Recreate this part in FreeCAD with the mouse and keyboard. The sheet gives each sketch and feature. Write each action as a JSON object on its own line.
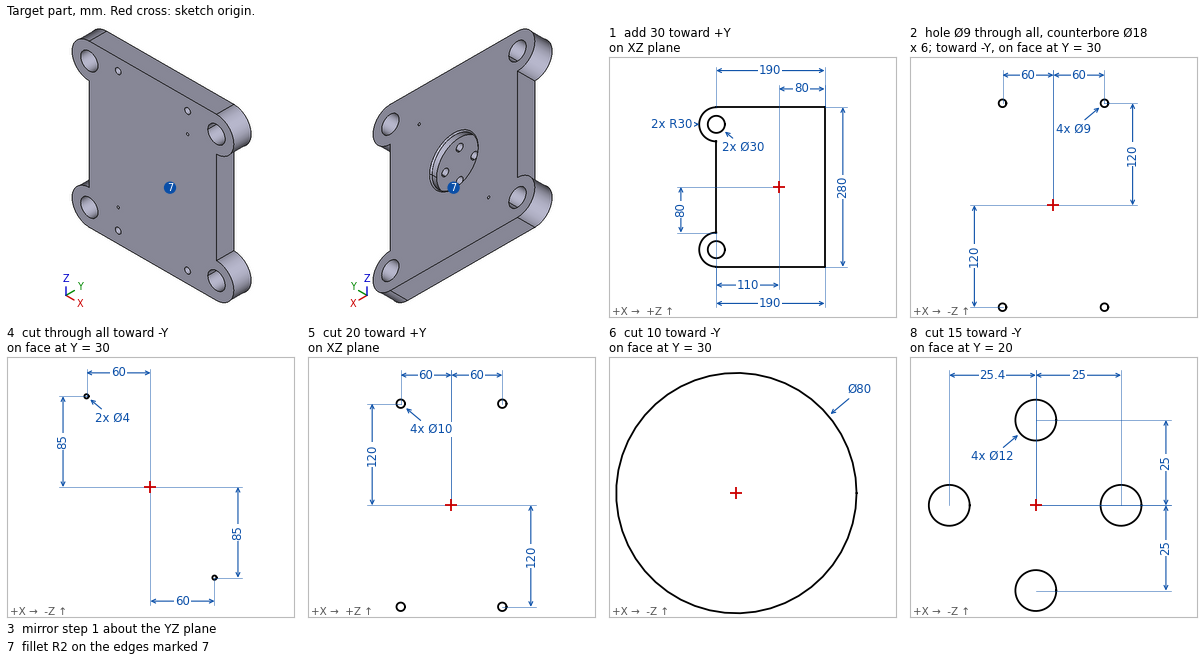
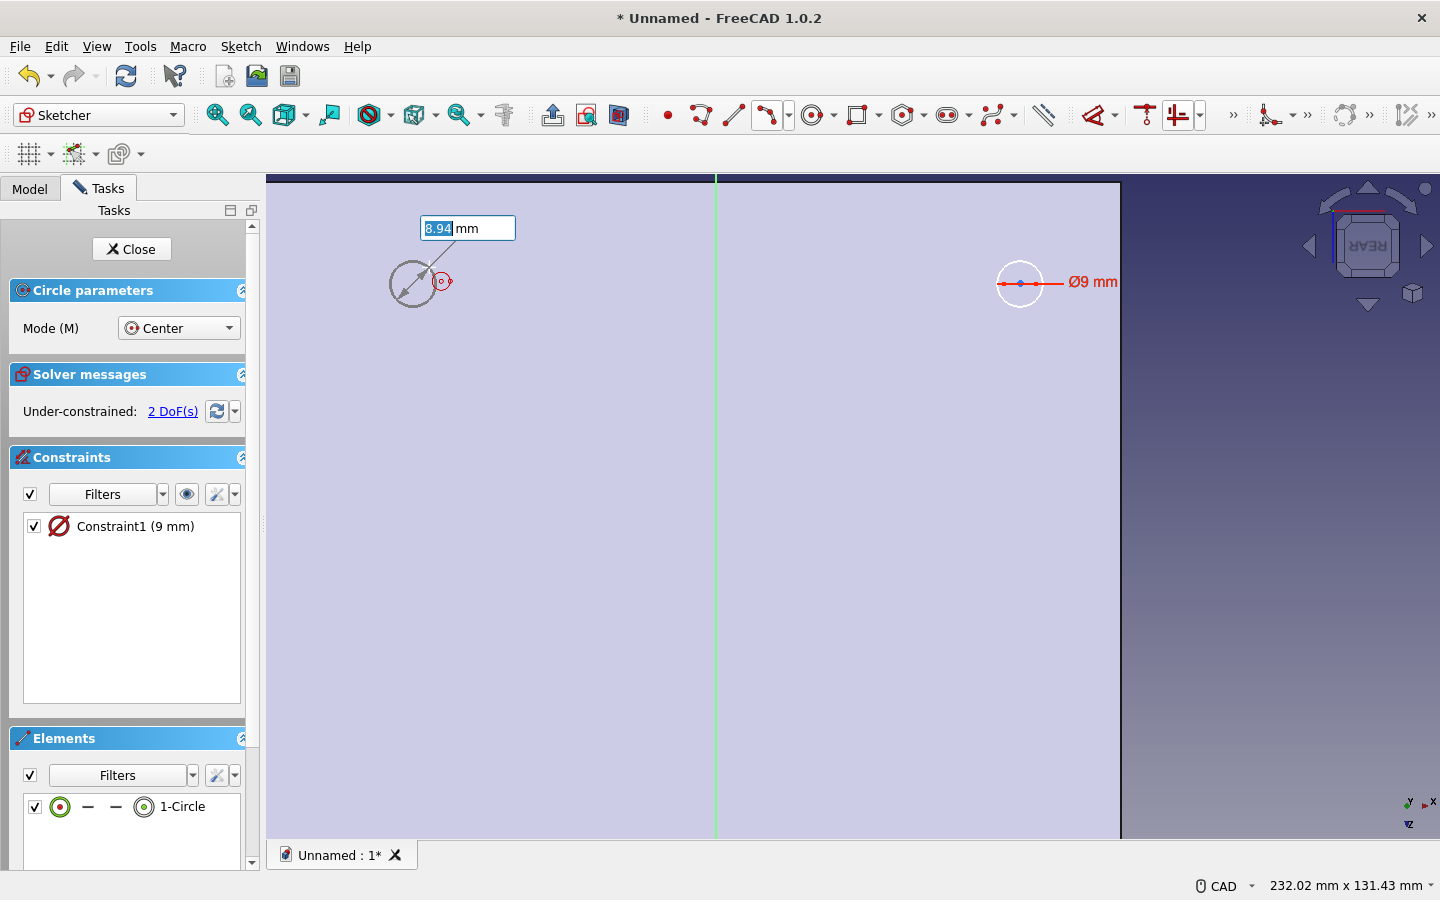
{"action": "type", "text": "9"}
{"action": "key", "text": "Return"}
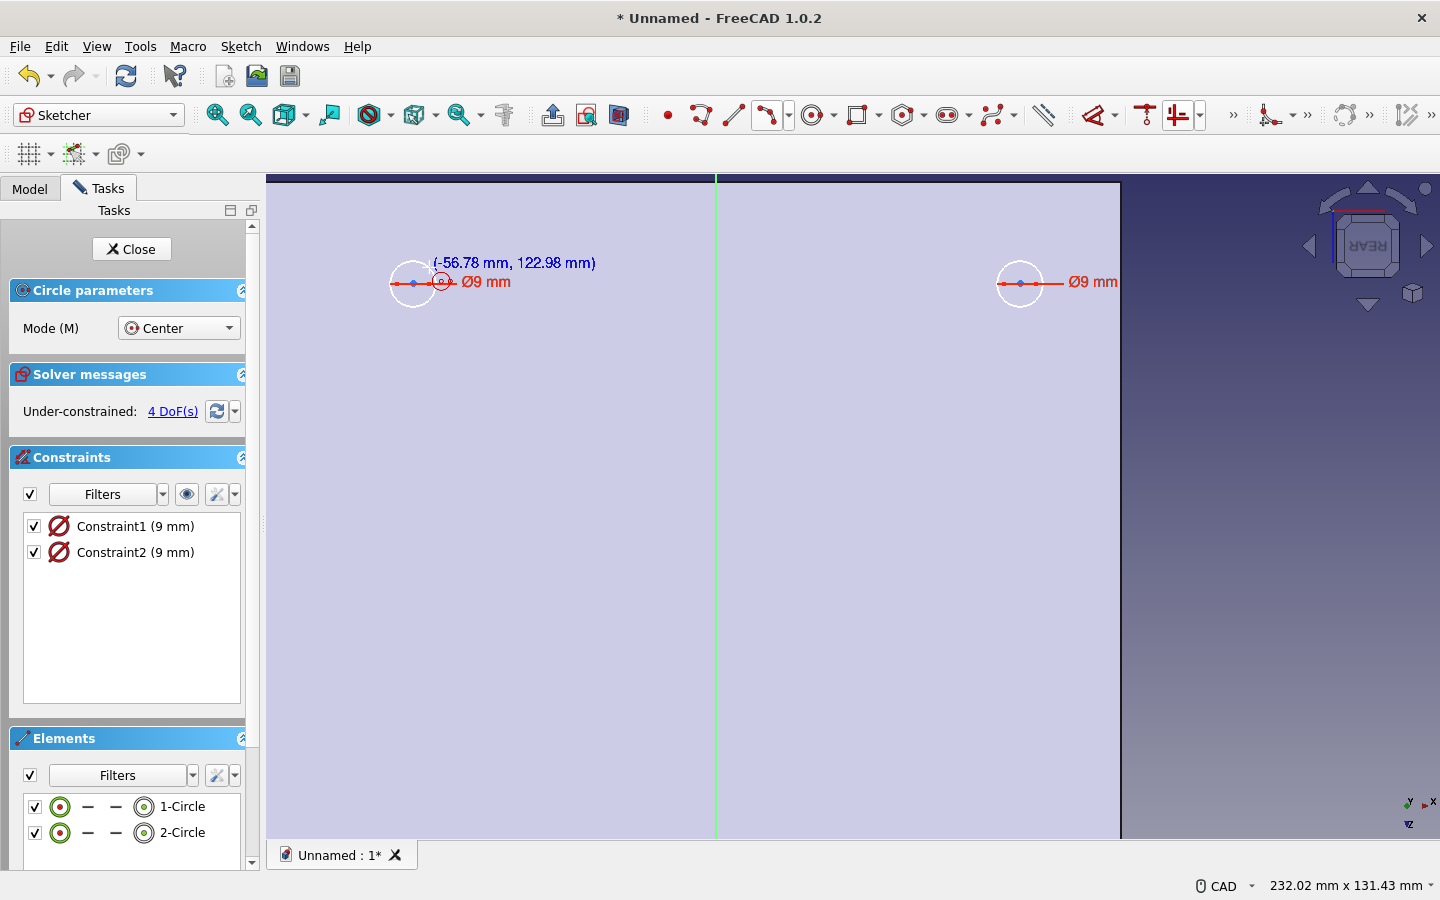
{"action": "scroll", "coordinate": [824, 283], "scroll_direction": "down", "scroll_amount": 5}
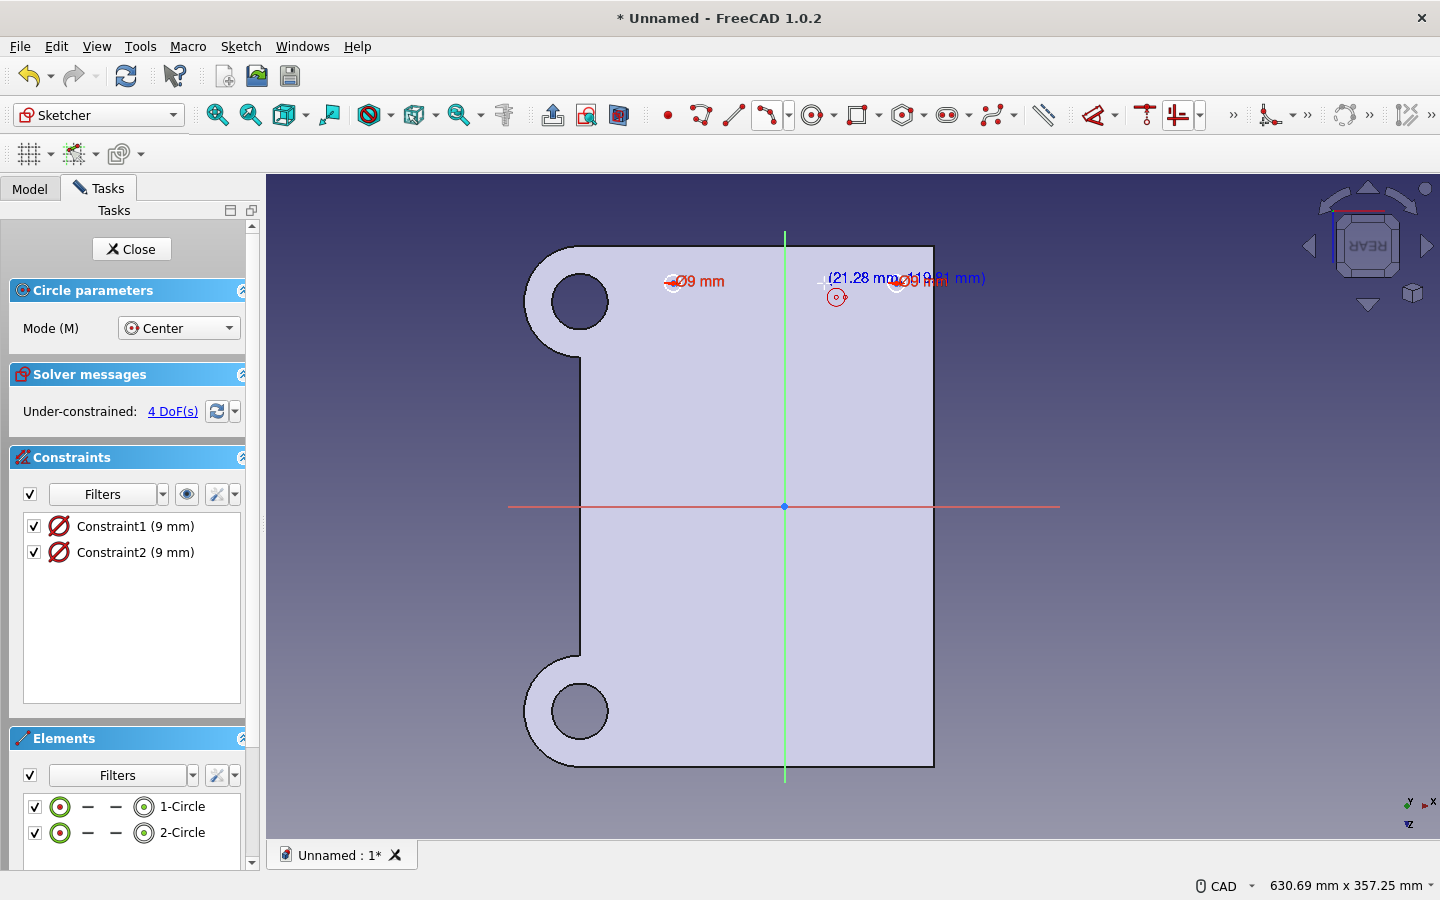
{"action": "scroll", "coordinate": [673, 730], "scroll_direction": "up", "scroll_amount": 5}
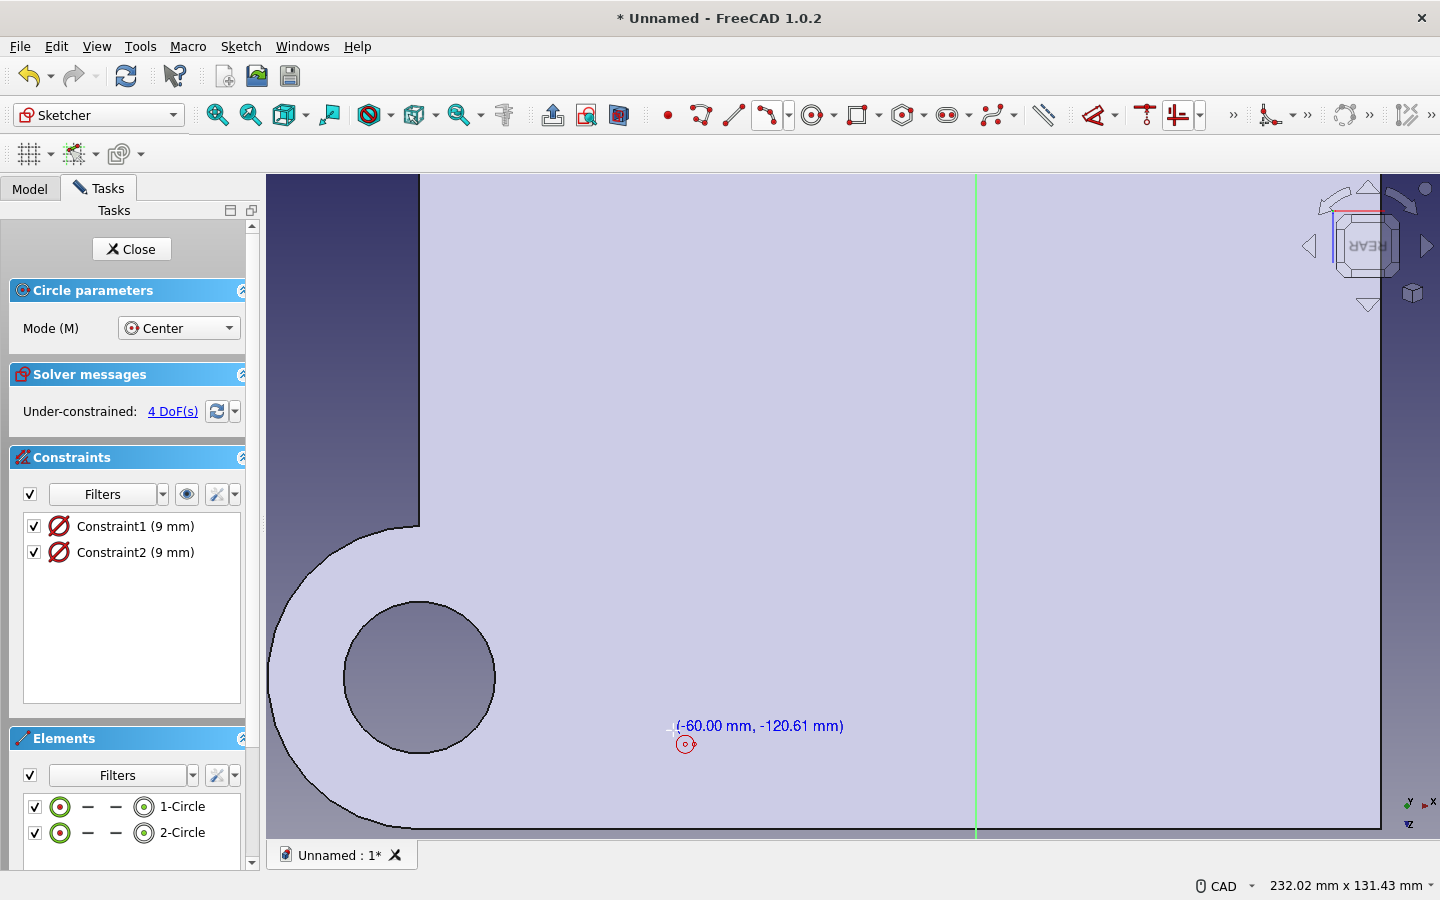
{"action": "left_click", "coordinate": [672, 728]}
{"action": "mouse_move", "coordinate": [689, 712]}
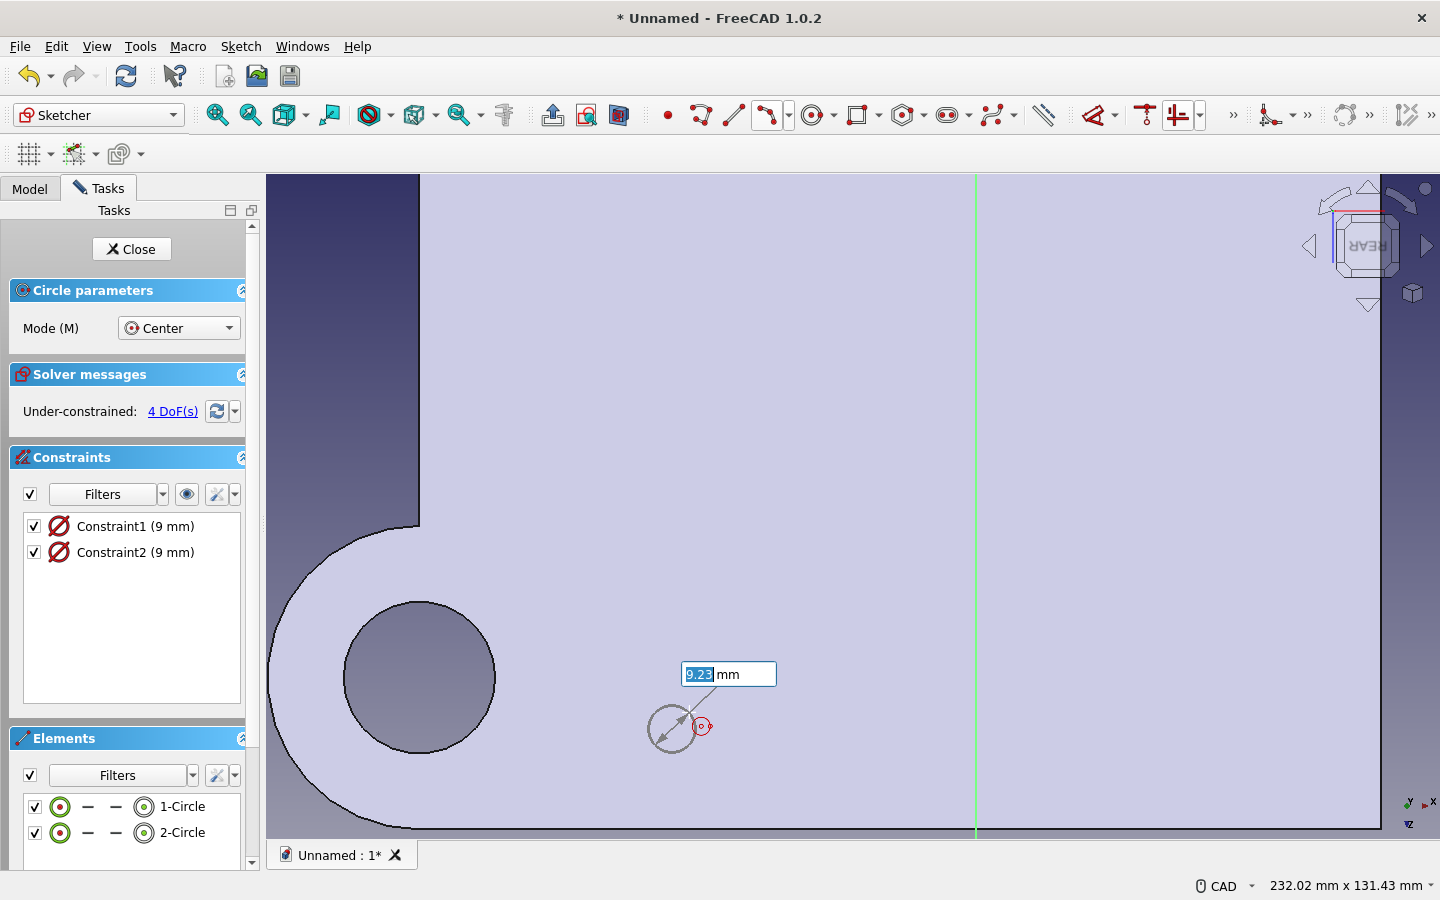
{"action": "type", "text": "9"}
{"action": "key", "text": "Return"}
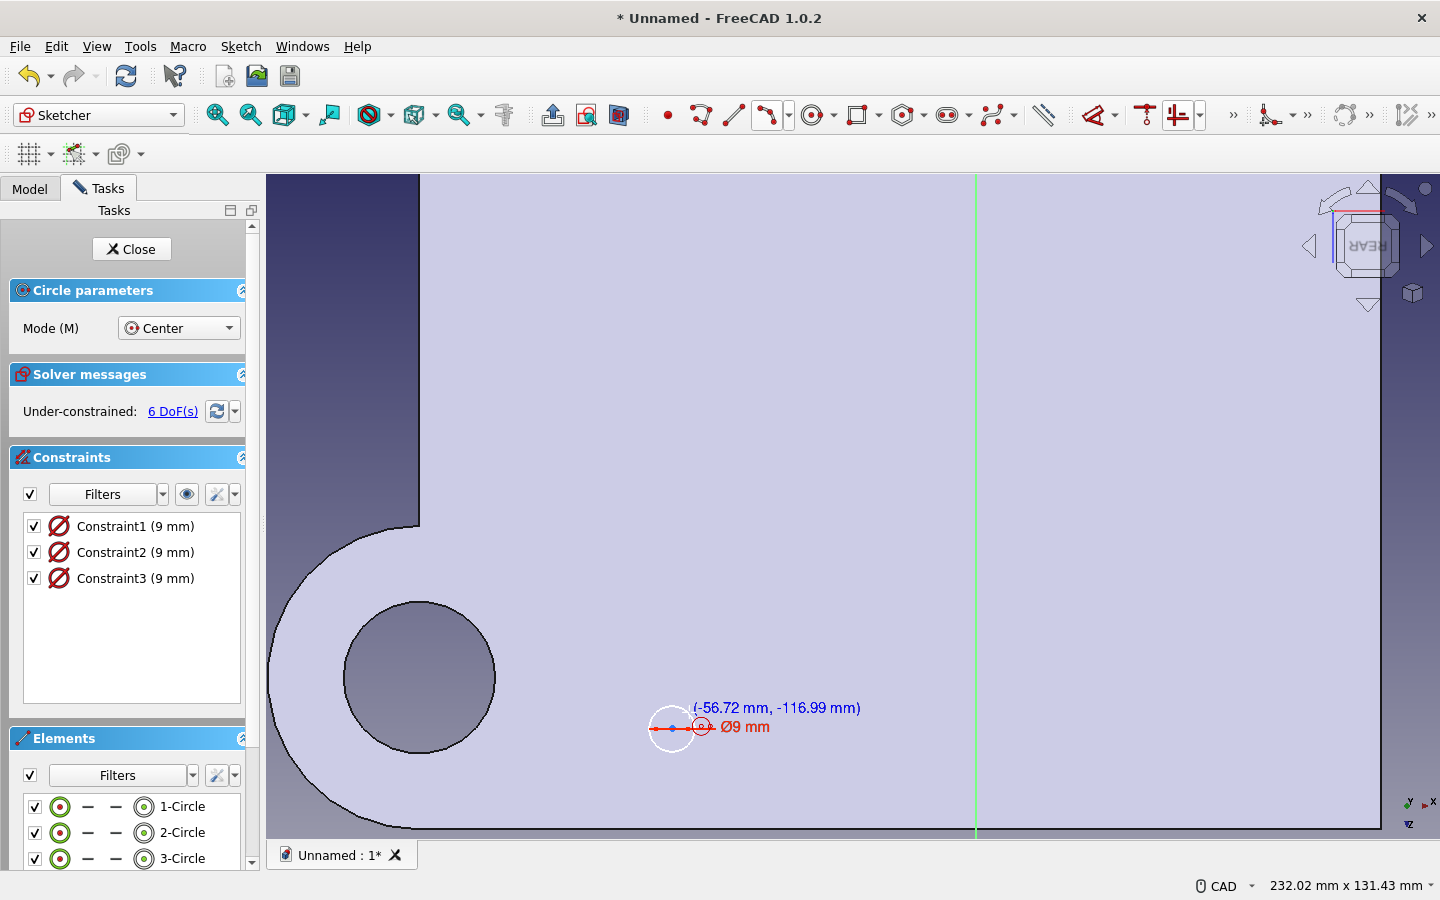
{"action": "scroll", "coordinate": [673, 731], "scroll_direction": "down", "scroll_amount": 5}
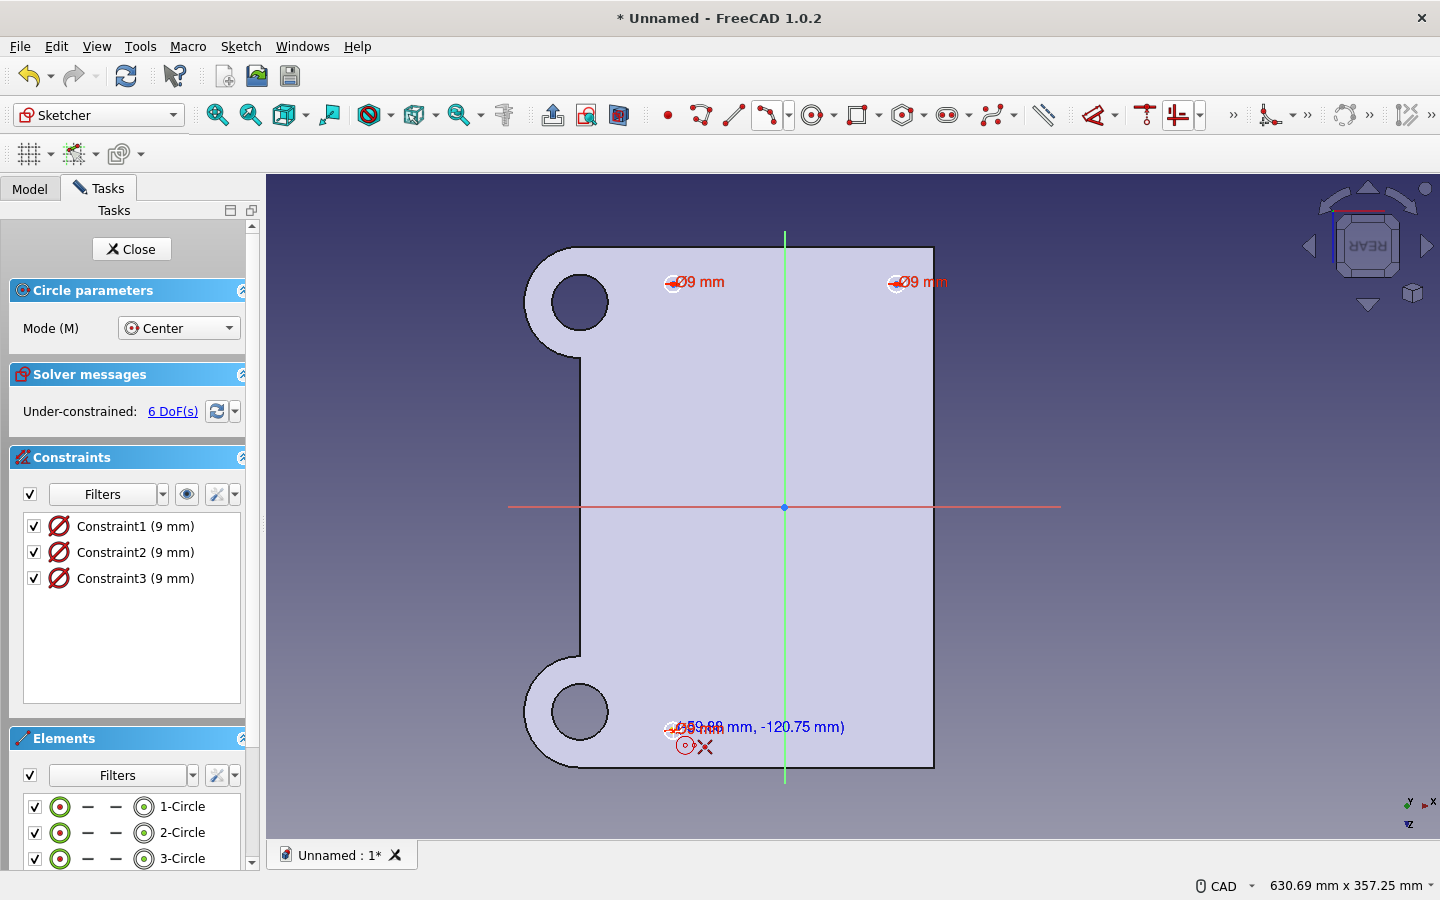
{"action": "scroll", "coordinate": [896, 731], "scroll_direction": "up", "scroll_amount": 5}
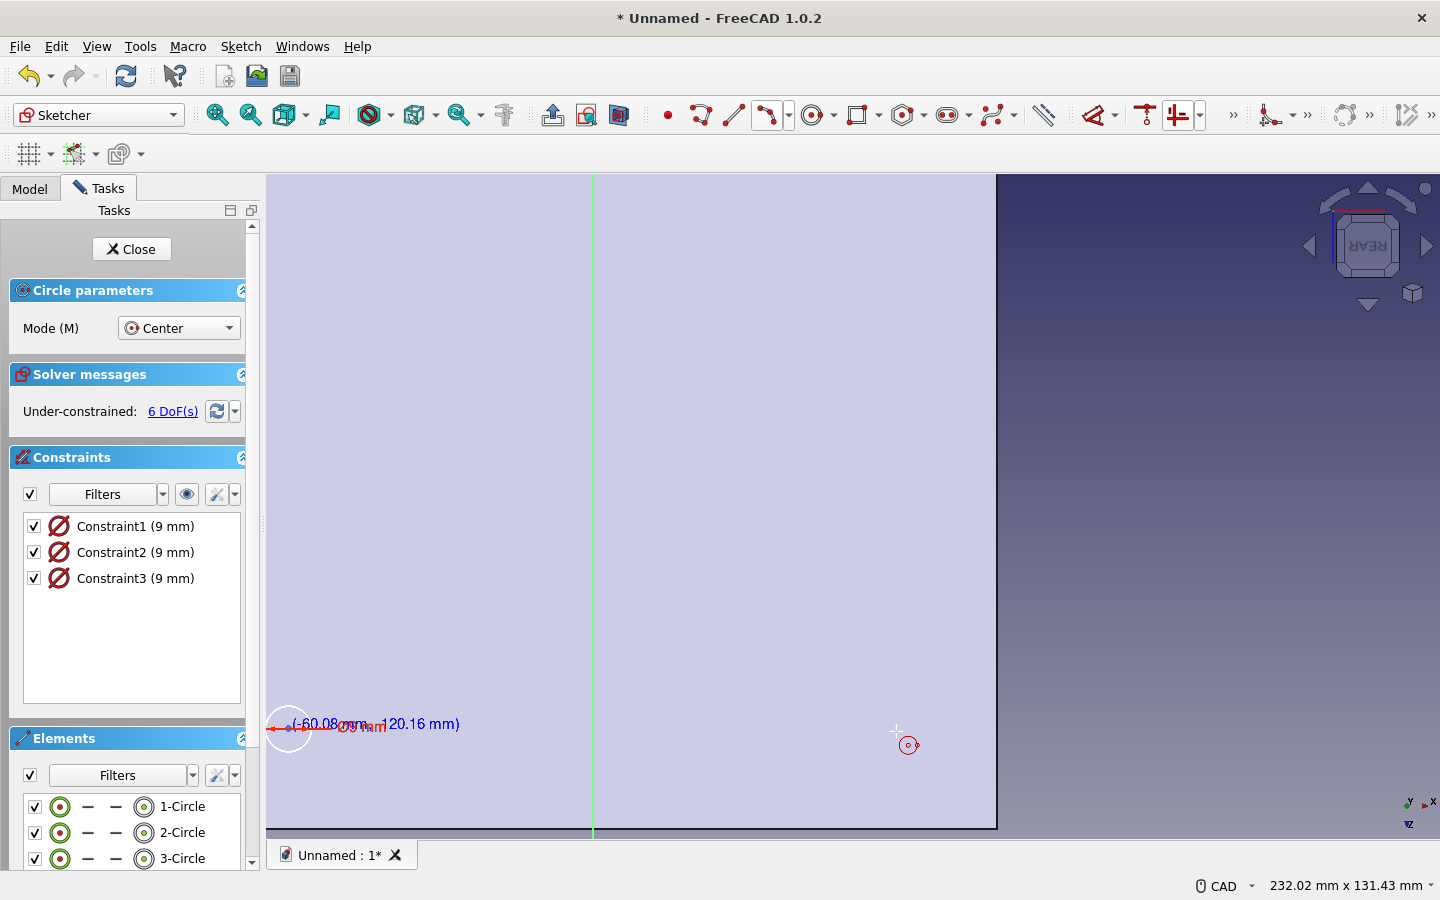
{"action": "left_click", "coordinate": [896, 728]}
{"action": "mouse_move", "coordinate": [912, 712]}